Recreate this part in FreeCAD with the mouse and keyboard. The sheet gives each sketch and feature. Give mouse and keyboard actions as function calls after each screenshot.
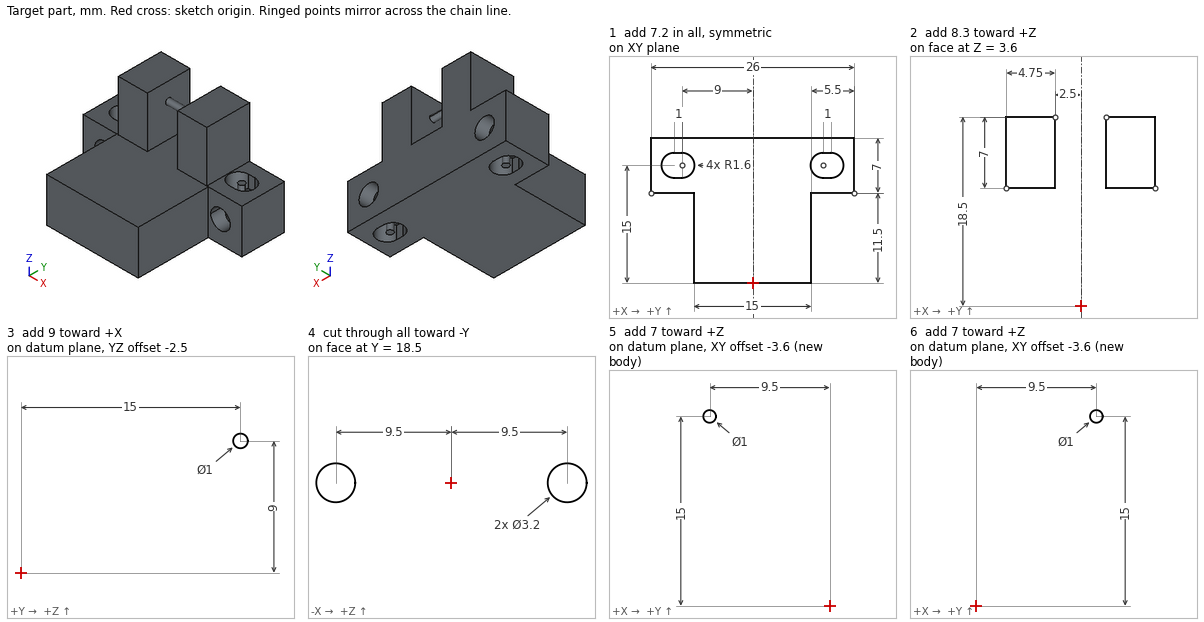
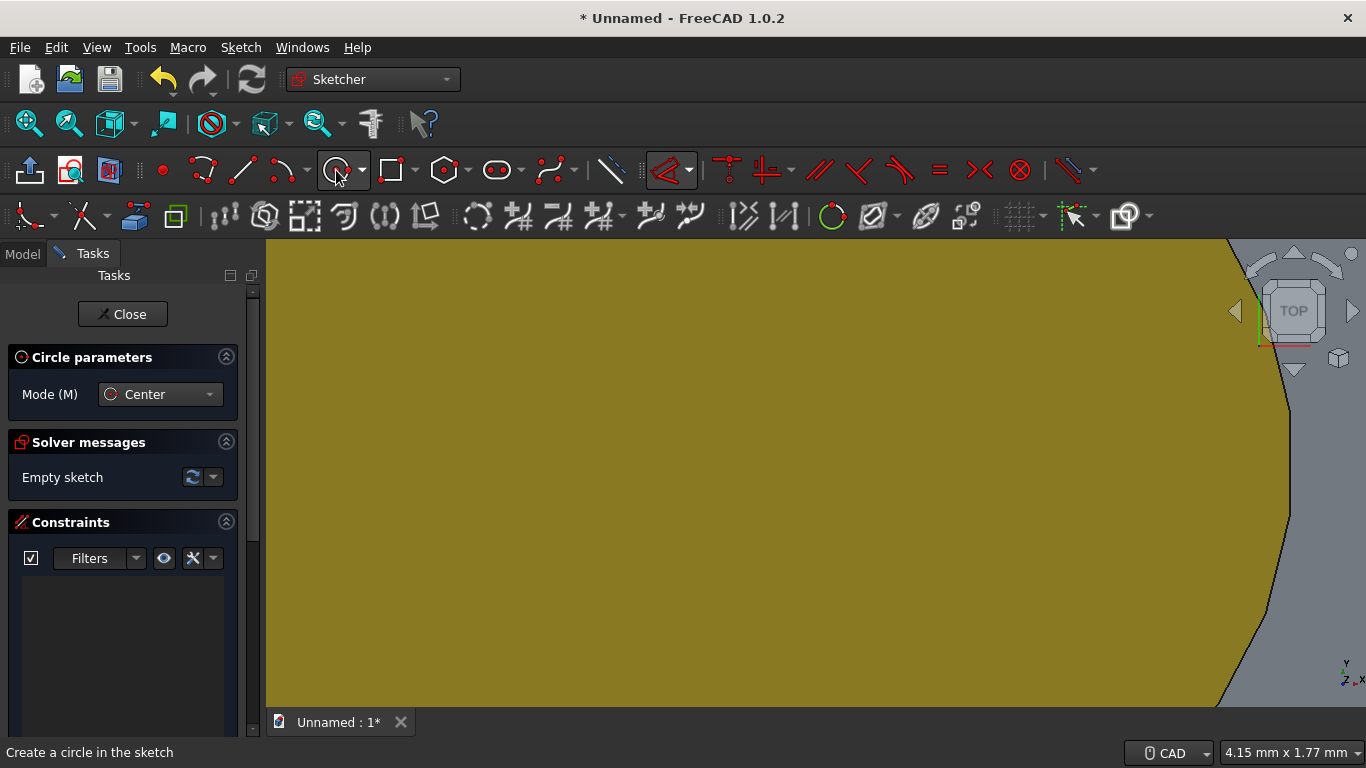
click(737, 463)
click(830, 370)
key(Escape)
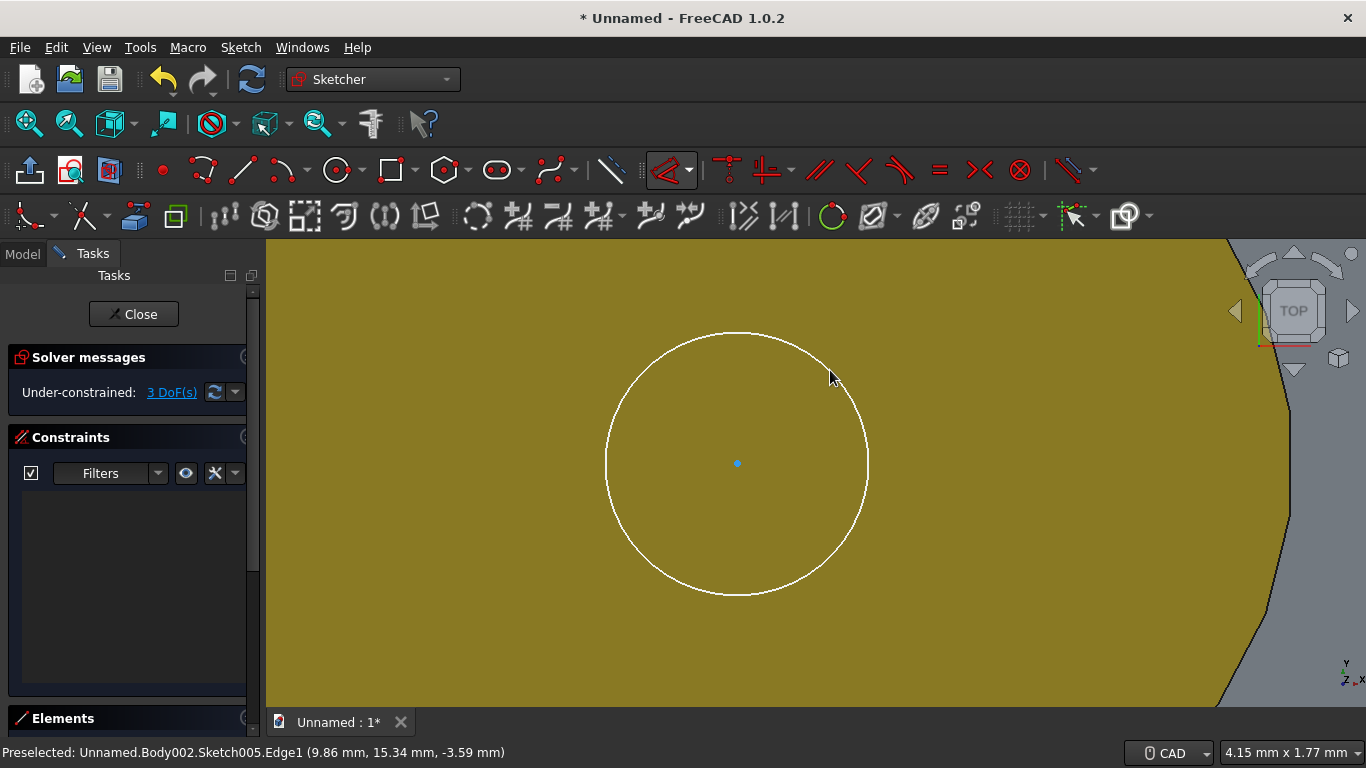
click(830, 371)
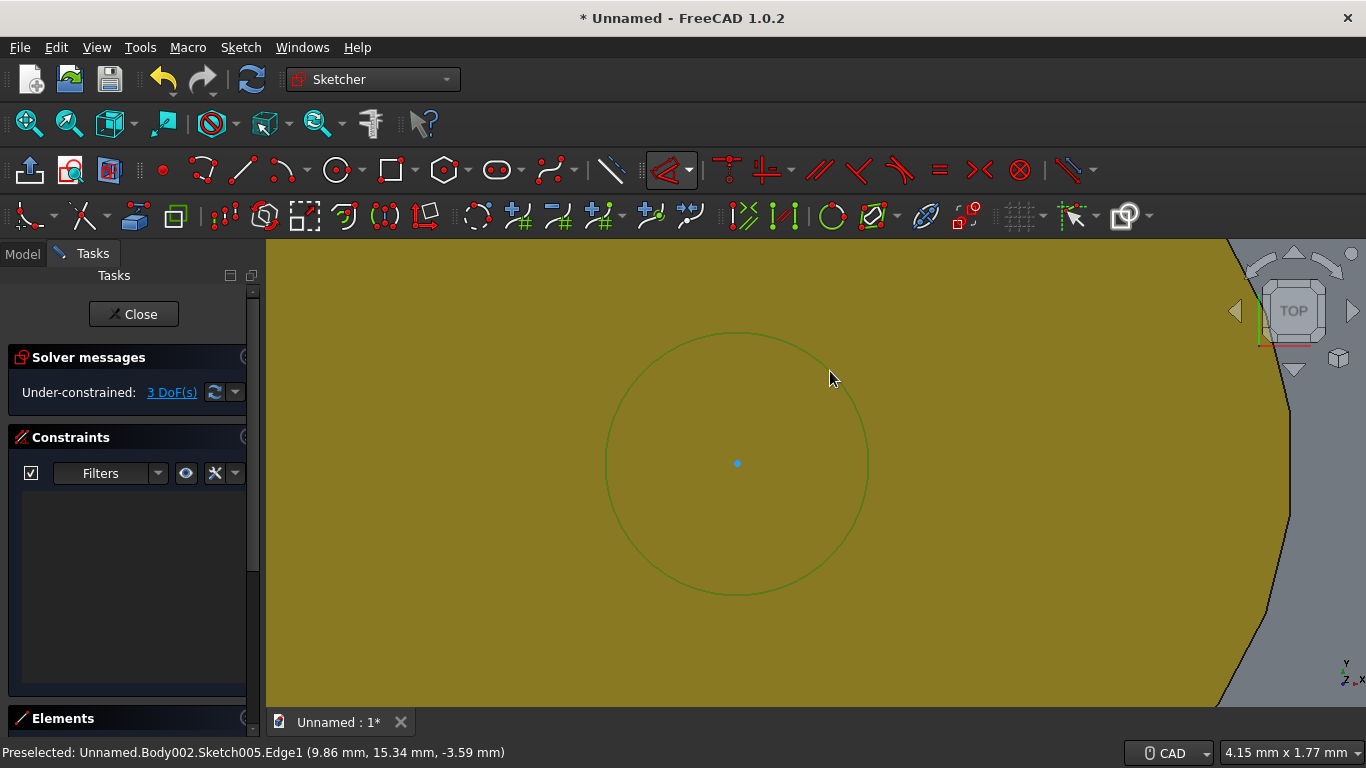
key(k)
key(o)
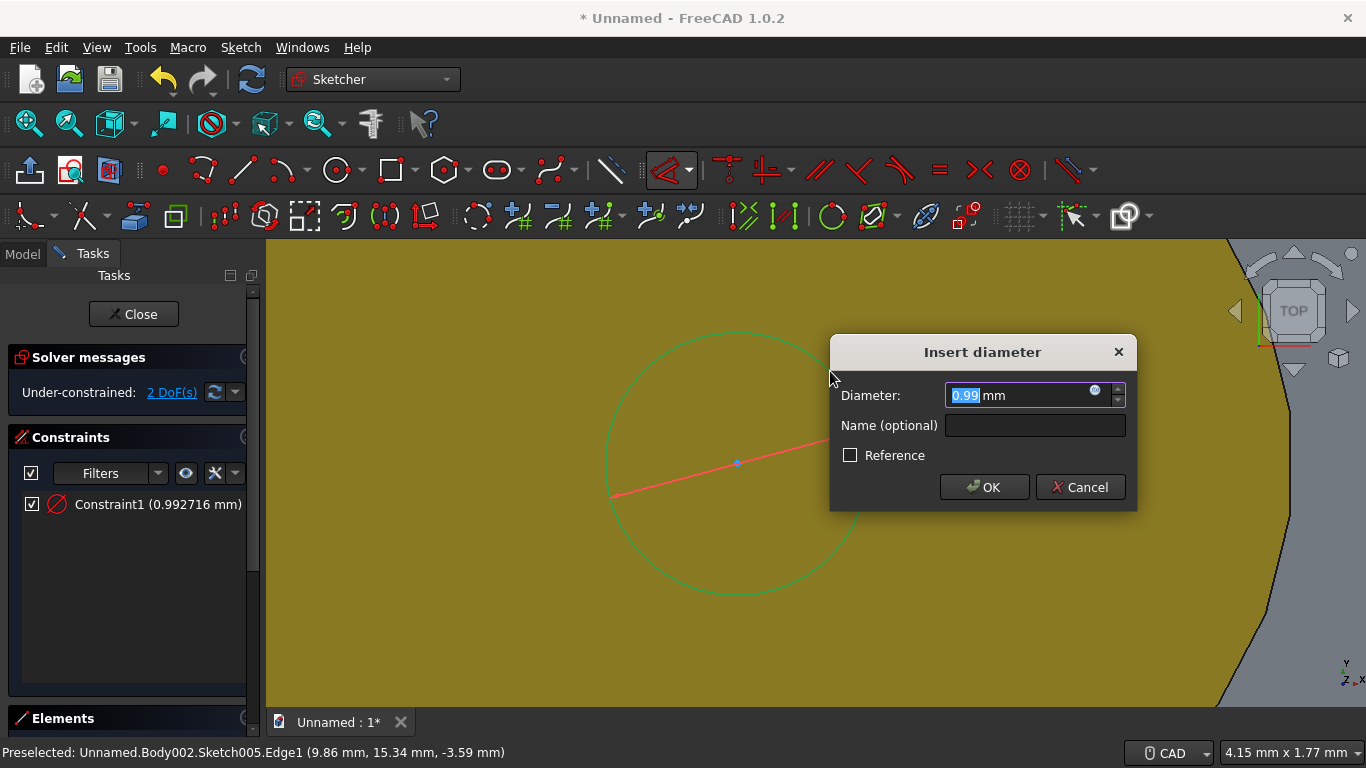
text(1)
key(Return)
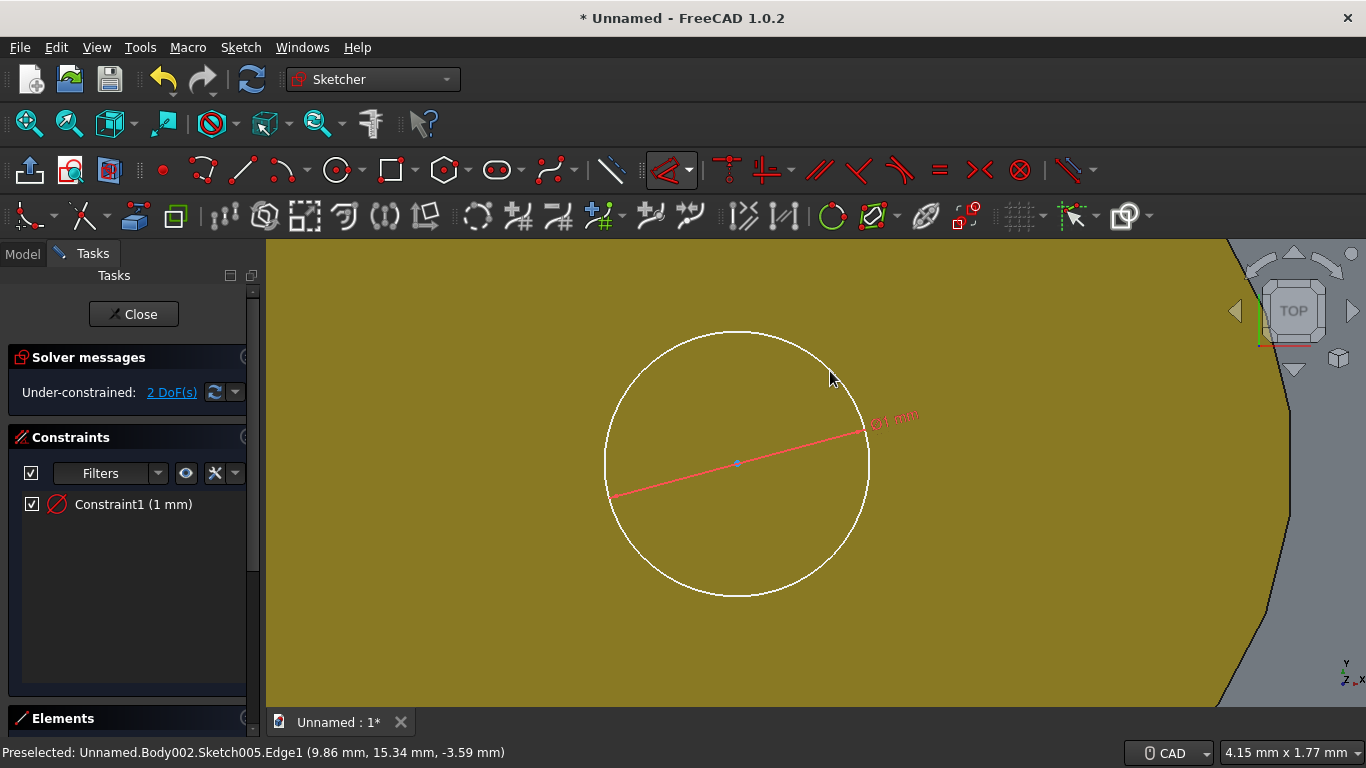
click(737, 464)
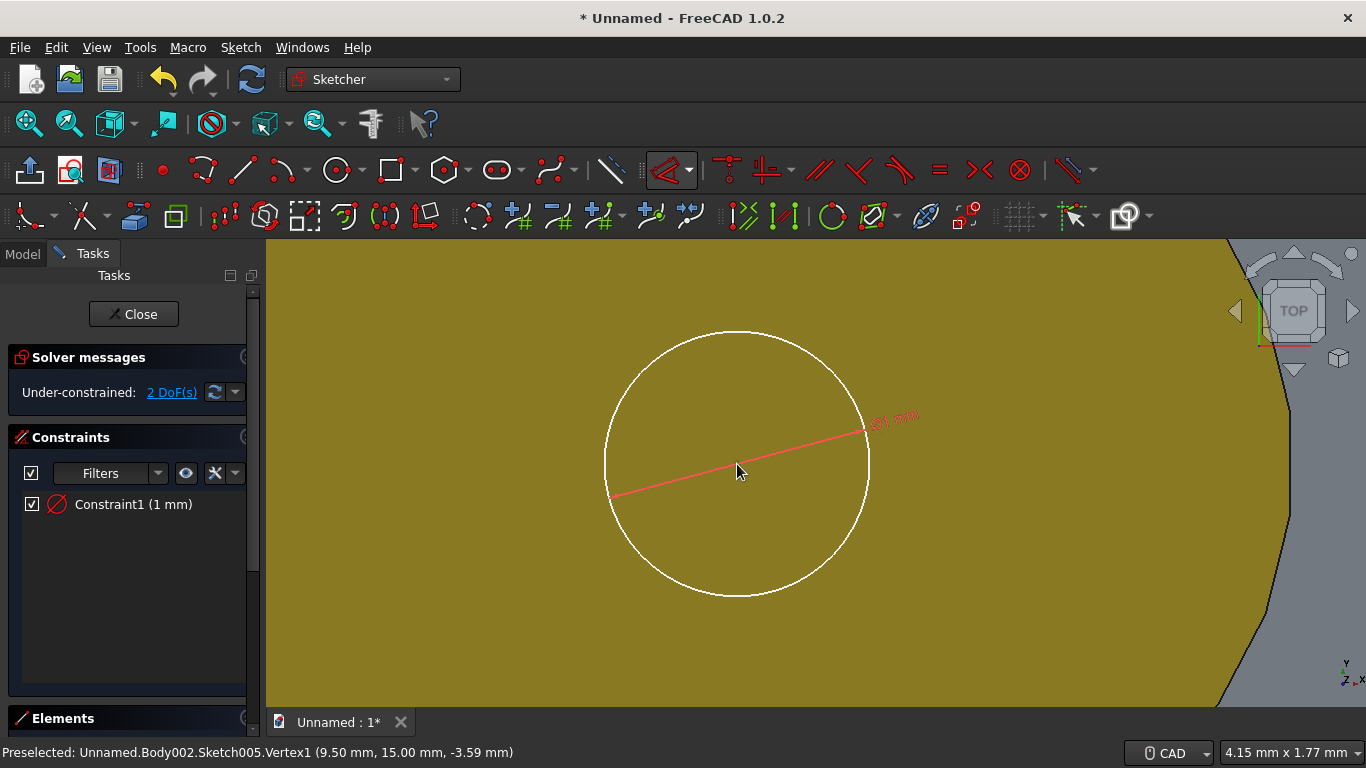
key(i)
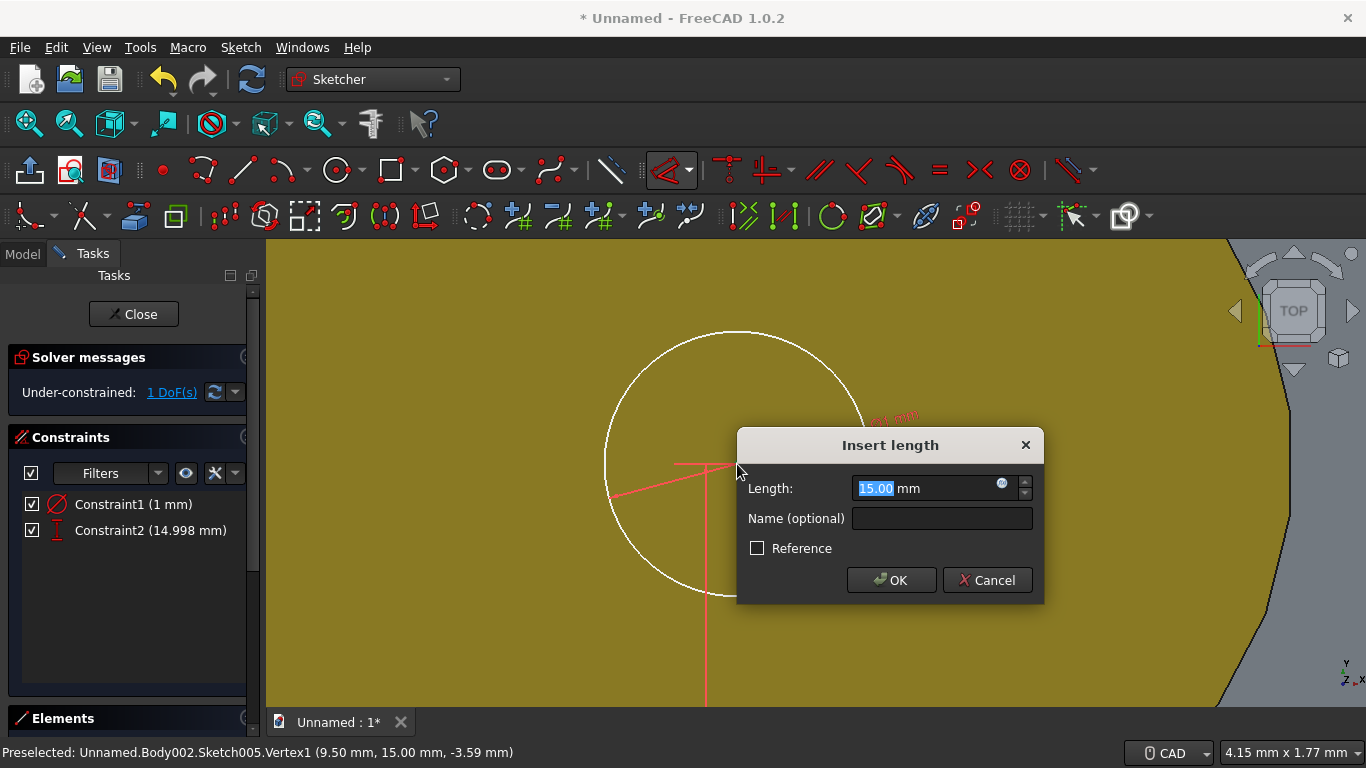
text(15)
key(Return)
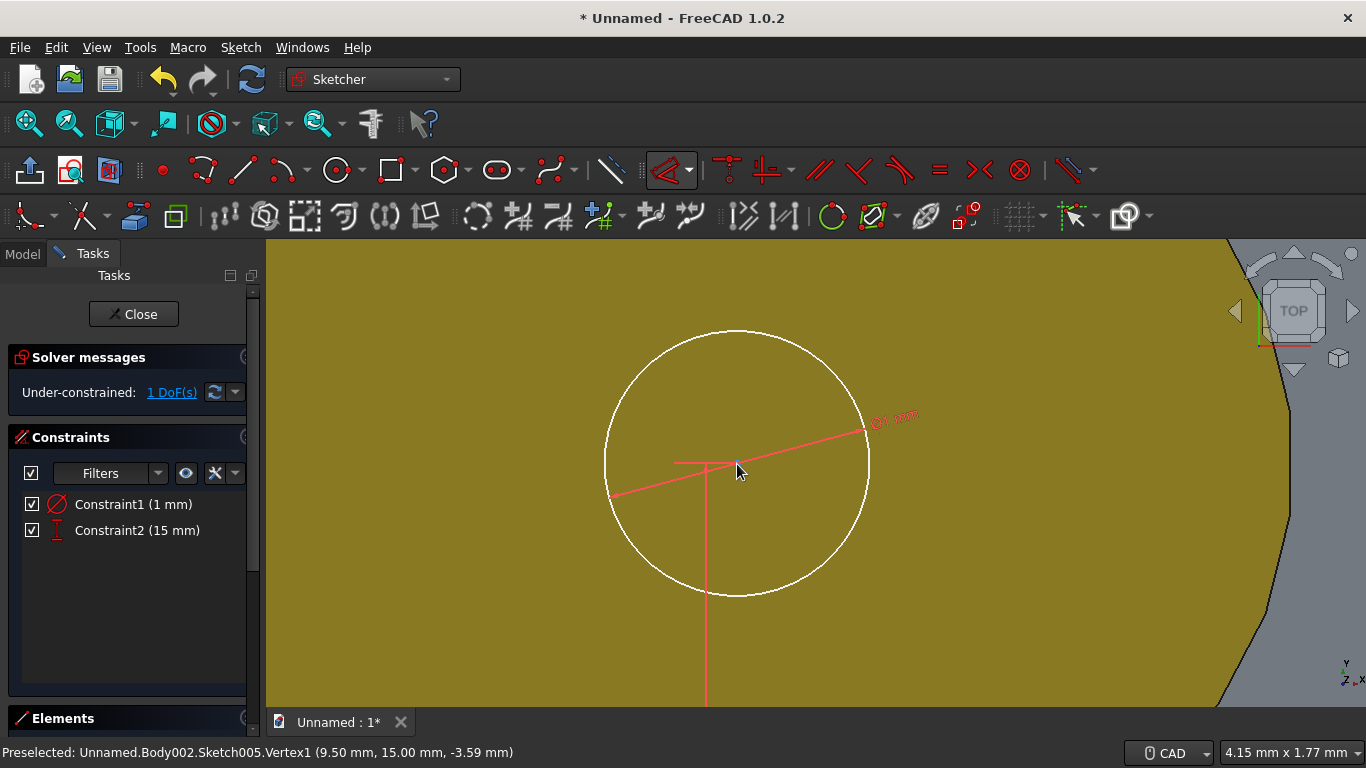
click(737, 463)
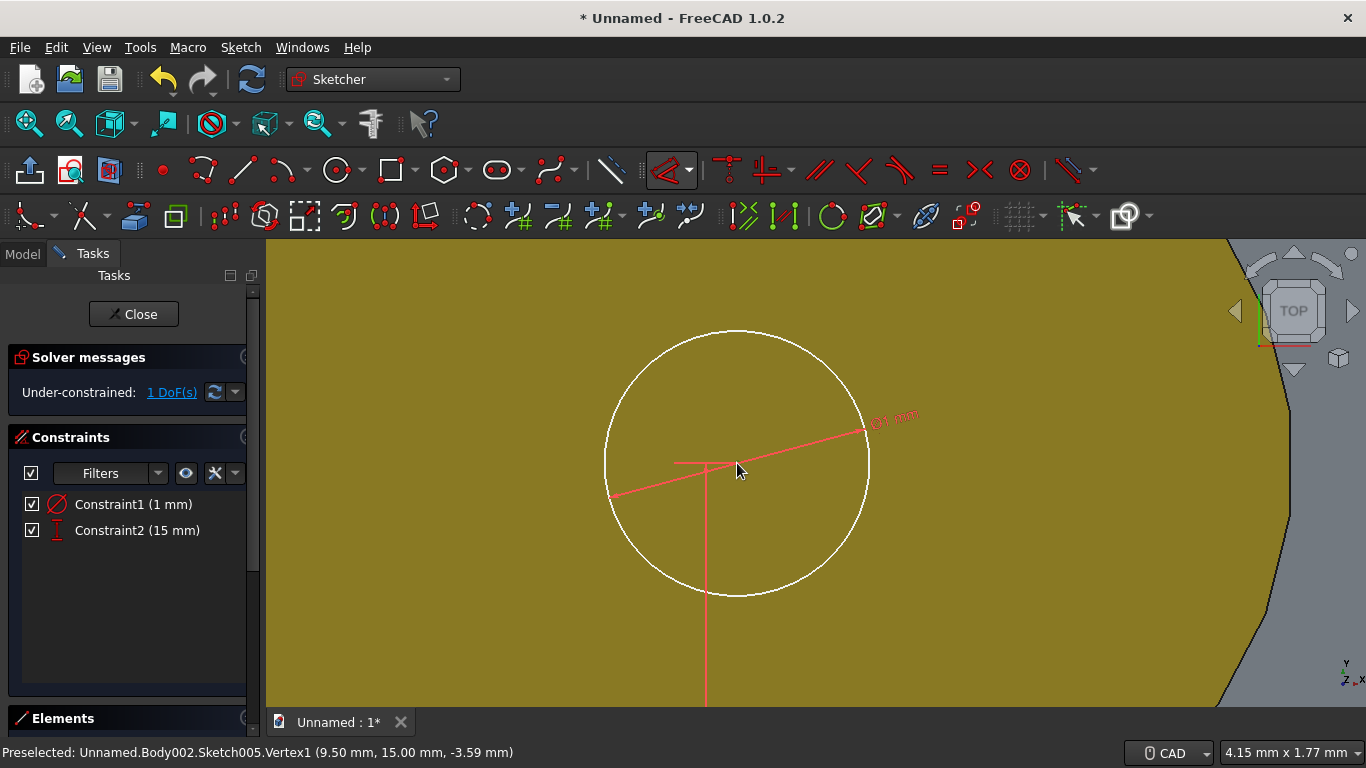
click(692, 170)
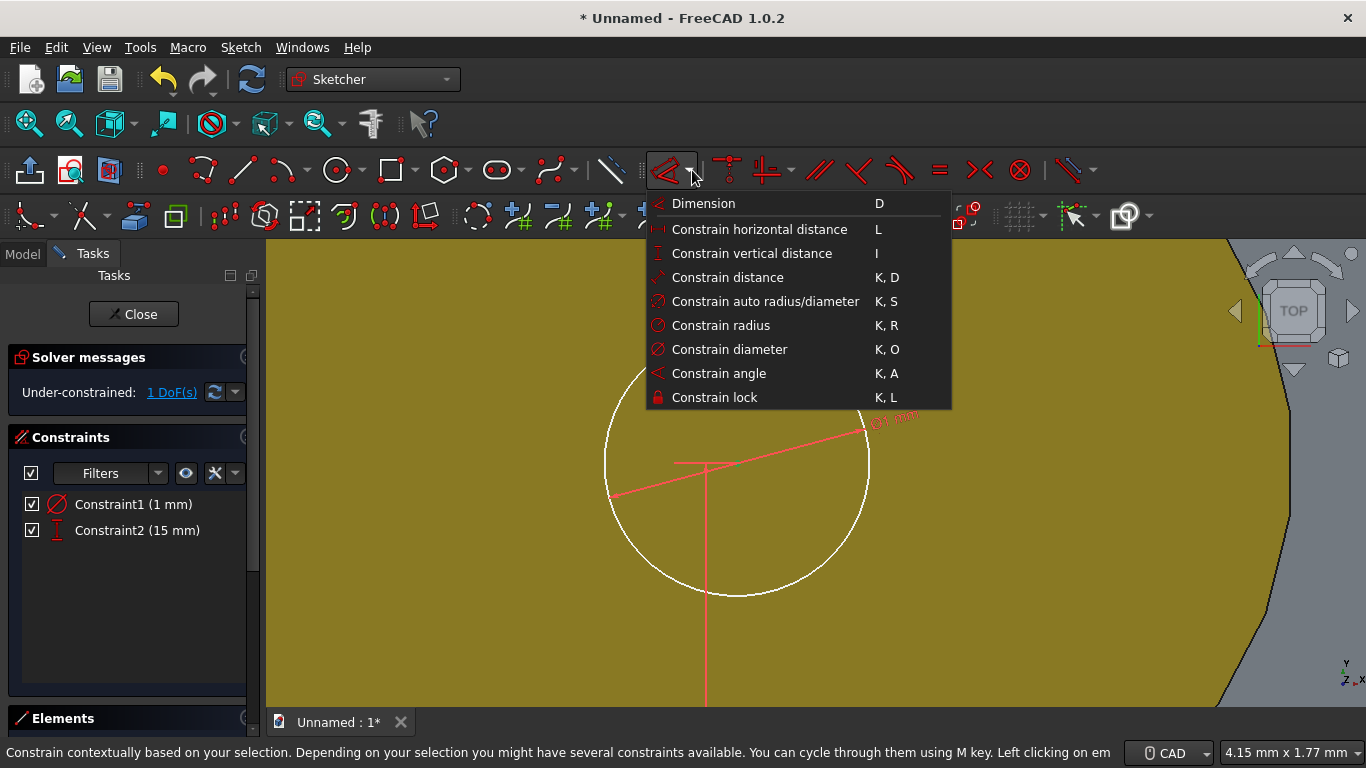
click(799, 229)